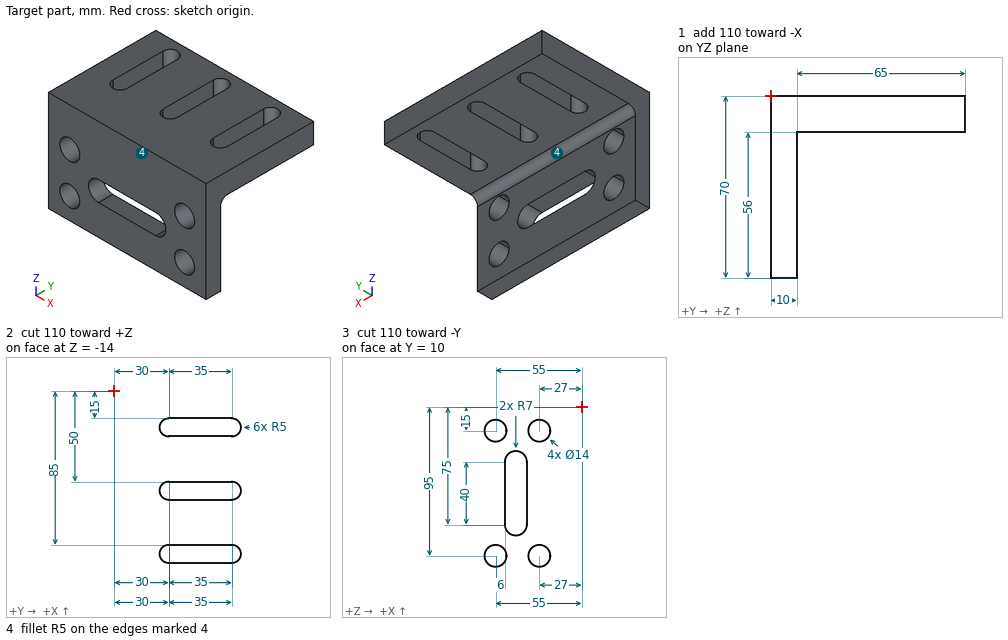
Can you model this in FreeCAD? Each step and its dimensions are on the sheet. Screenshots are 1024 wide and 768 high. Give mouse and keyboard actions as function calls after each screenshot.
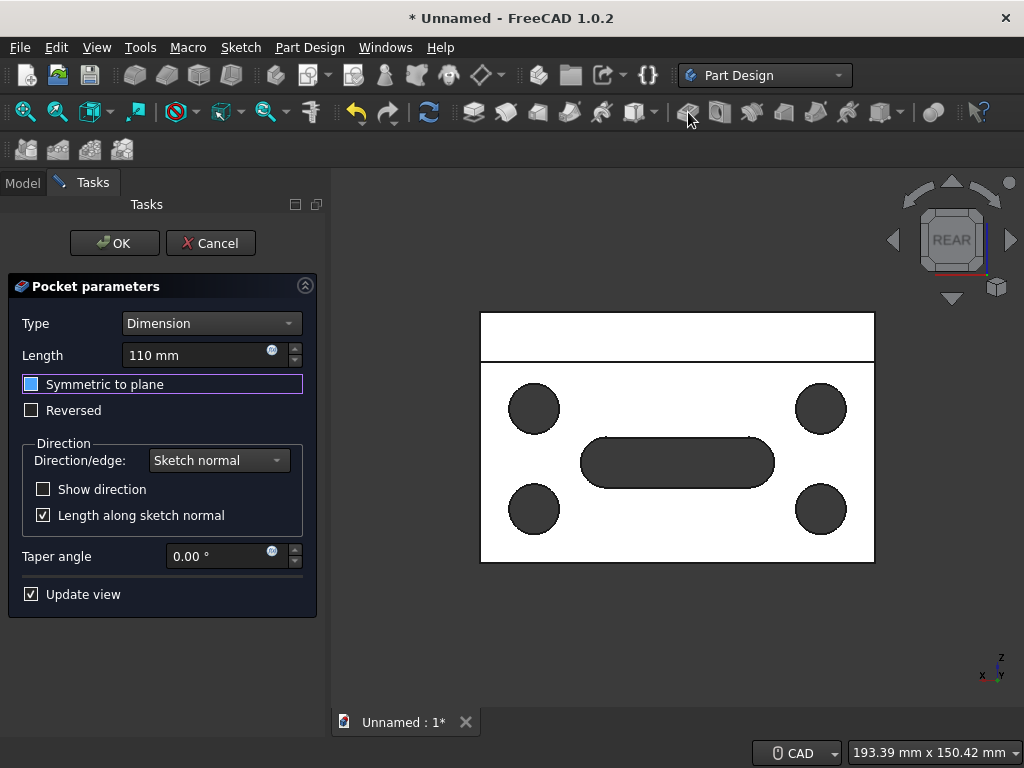
click(115, 243)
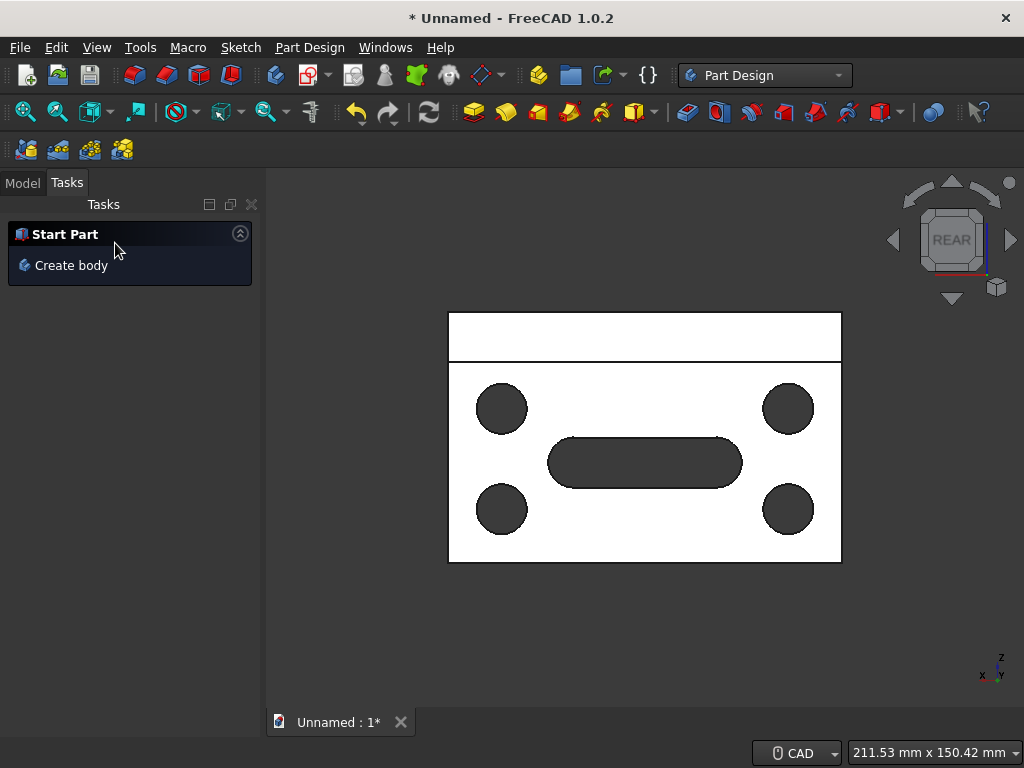
key(0)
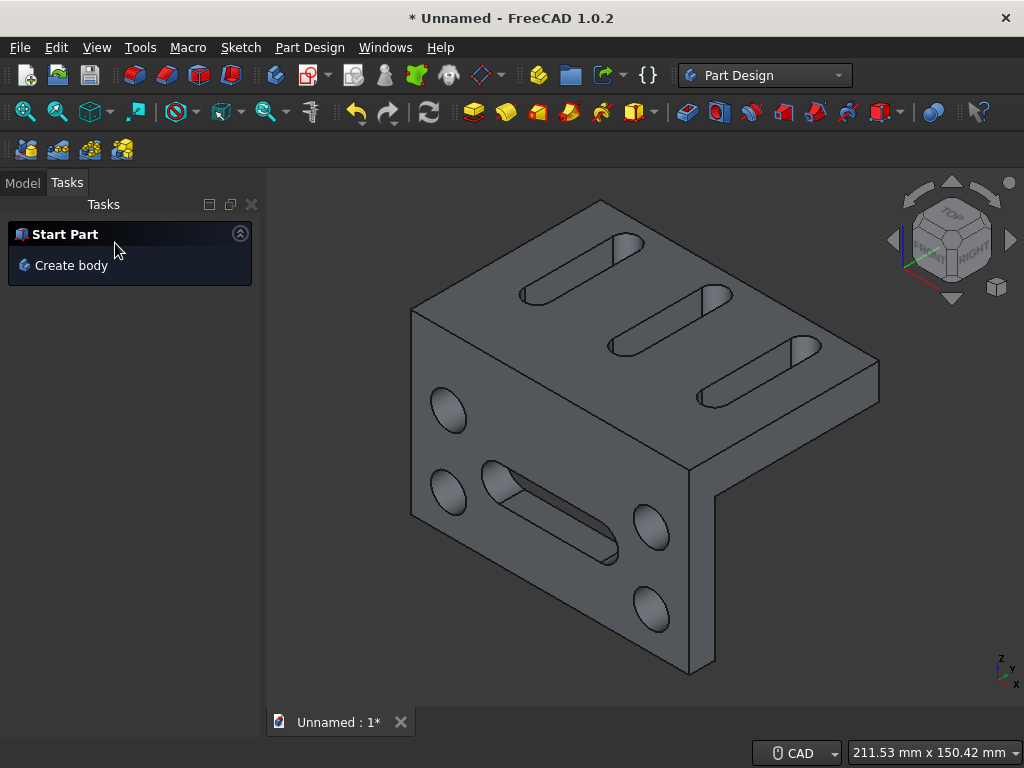
key(2)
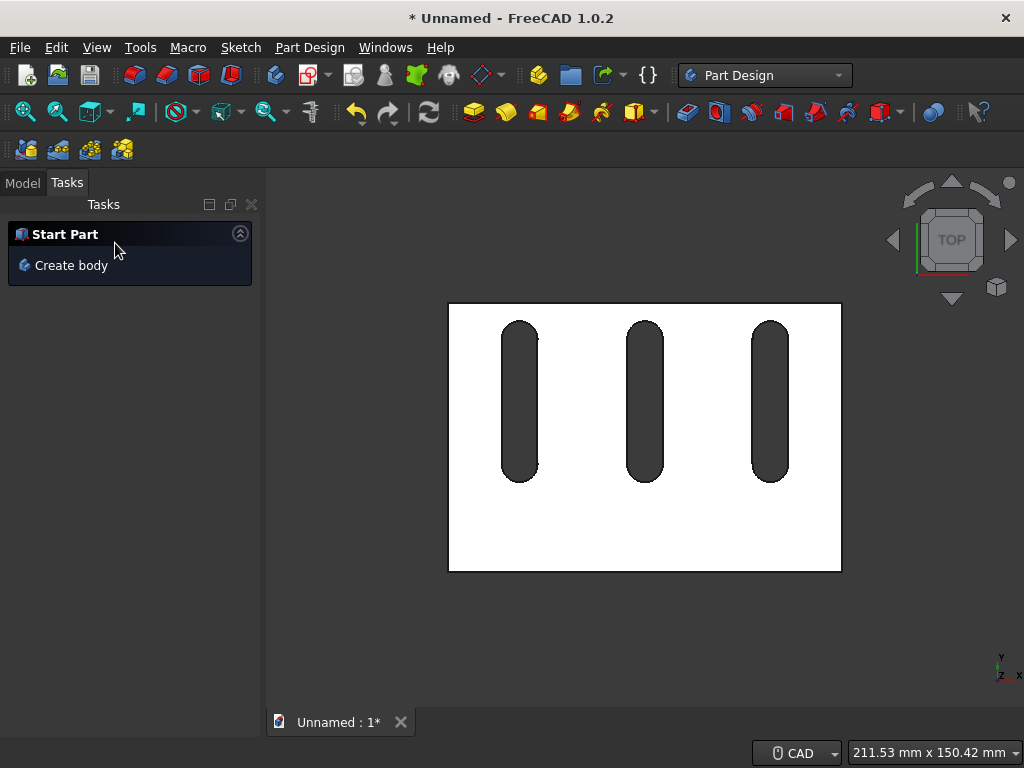
key(1)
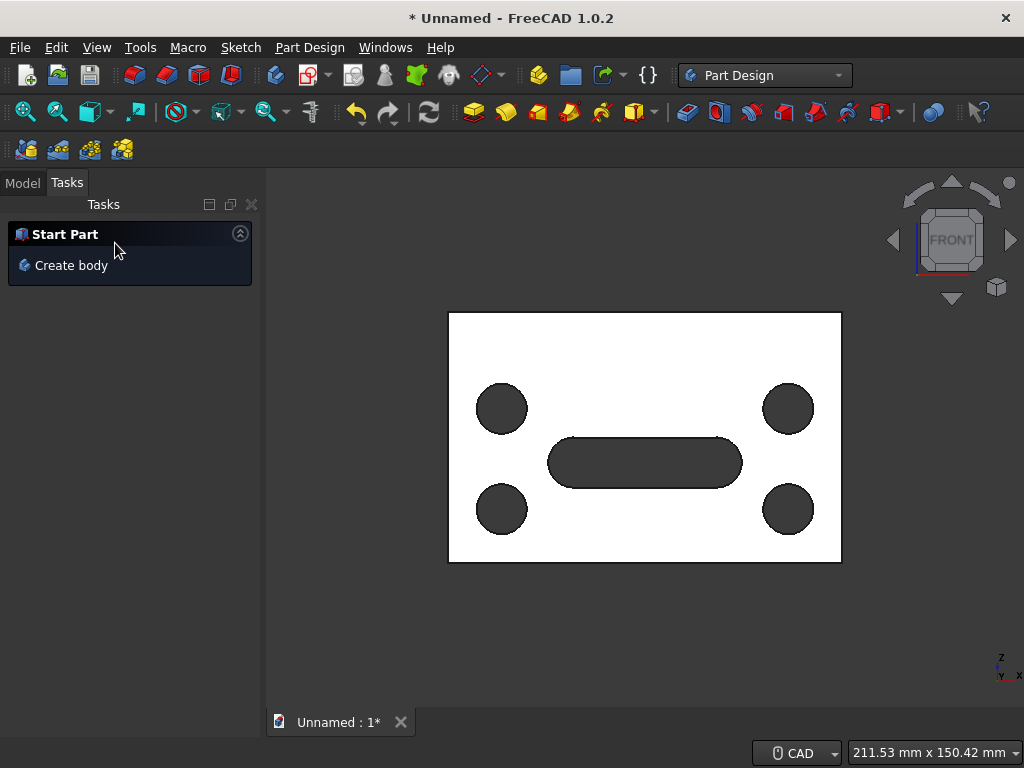
key(3)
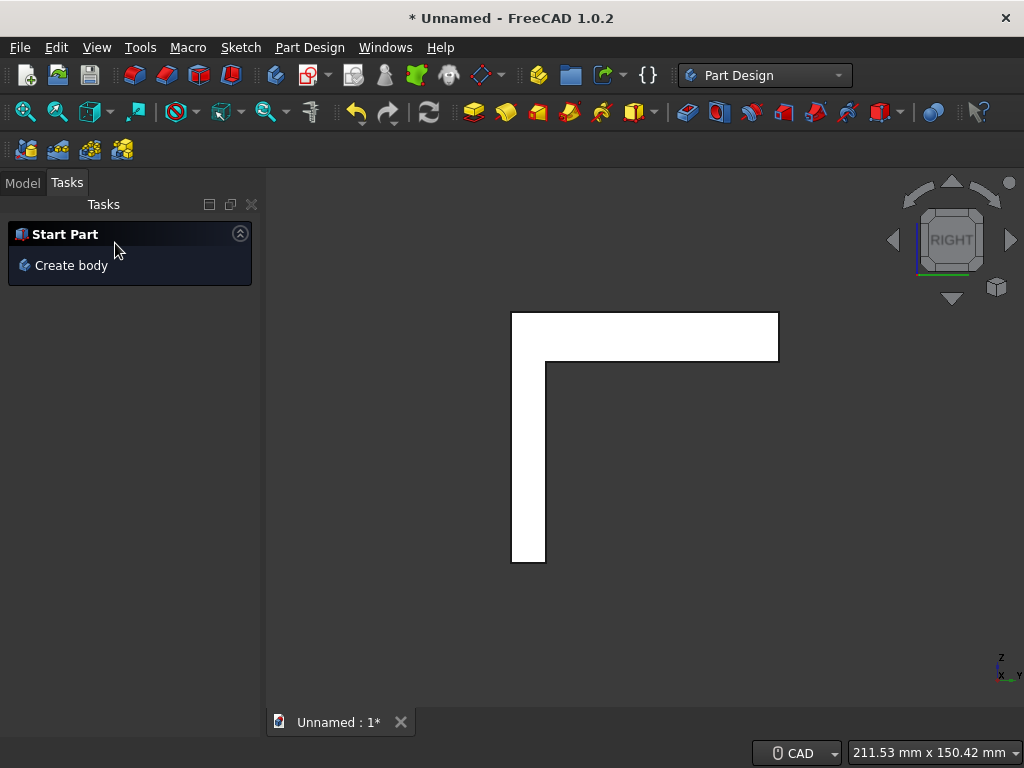
key(5)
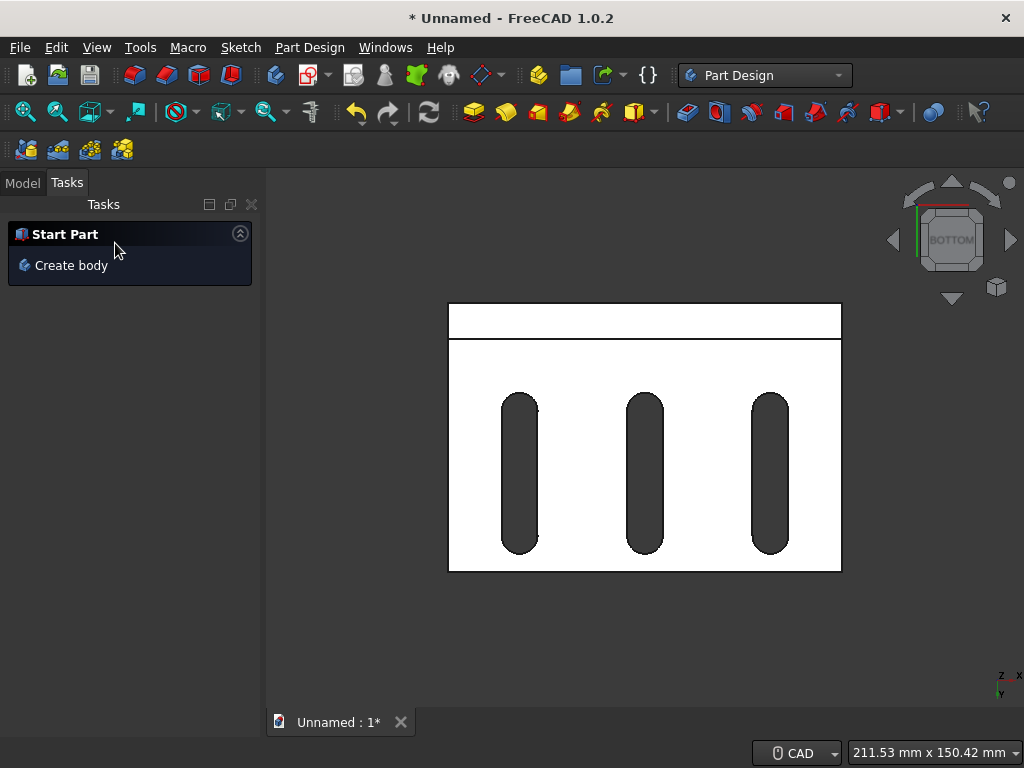
key(4)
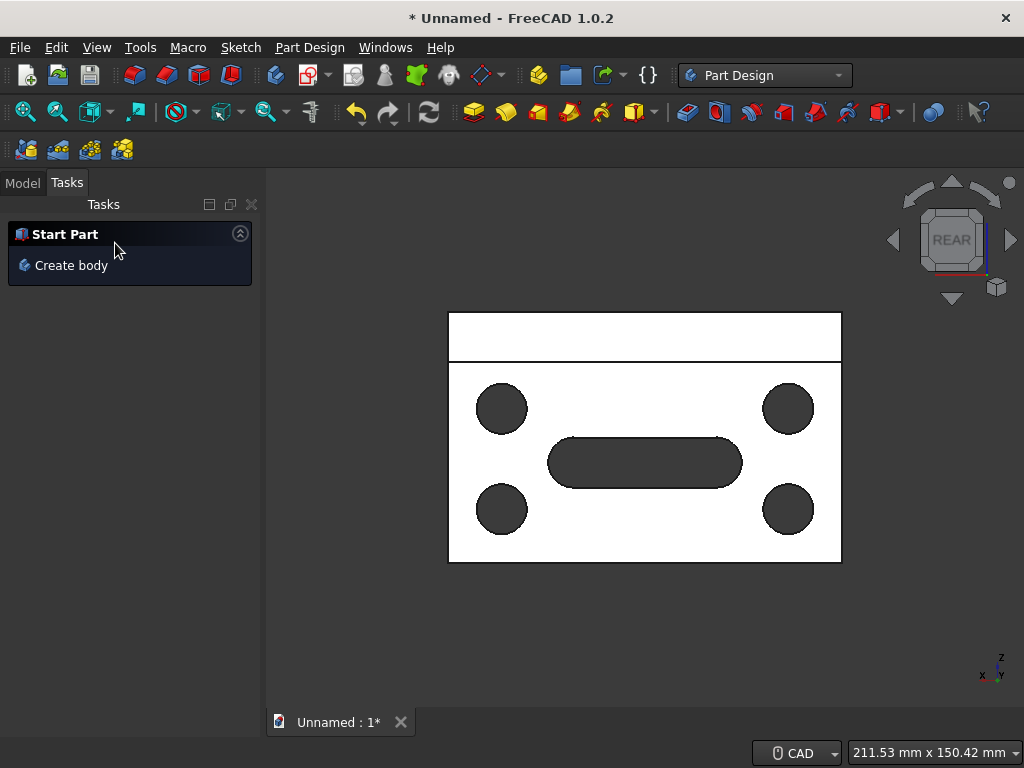
key(6)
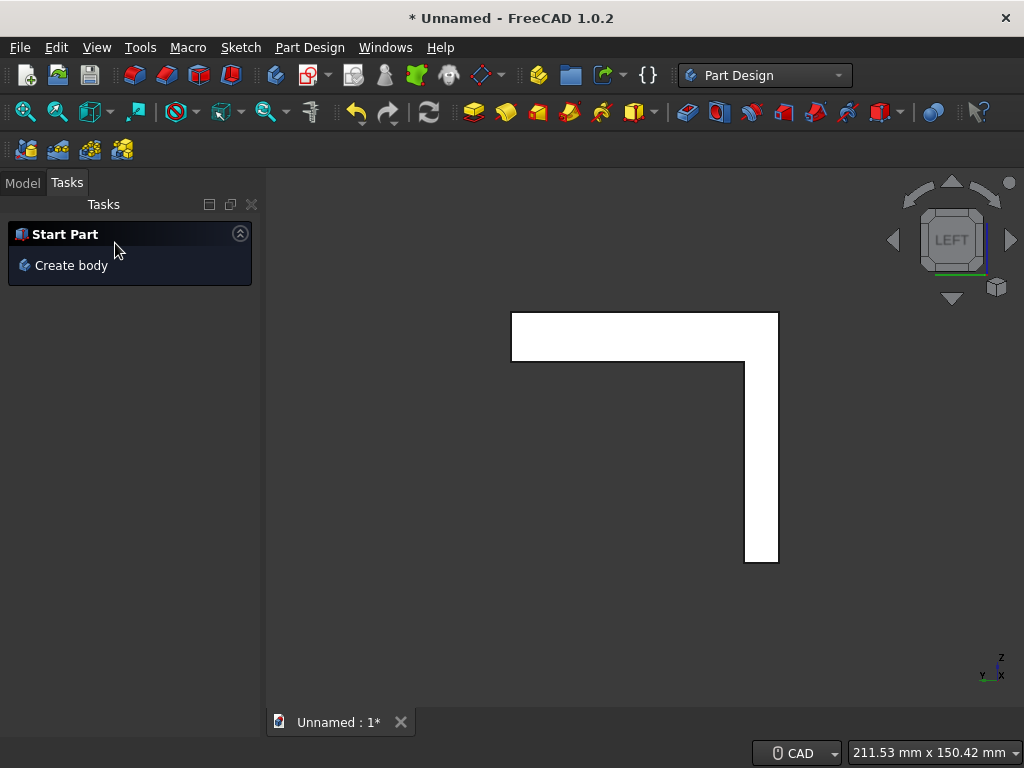
key(v)
key(3)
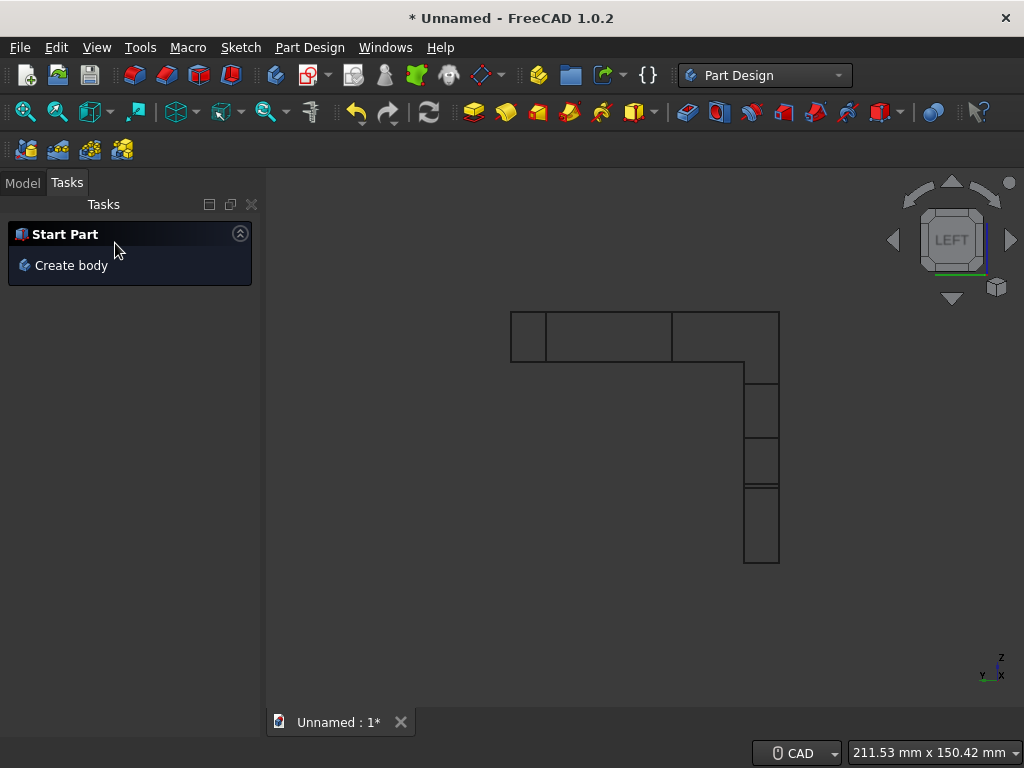
key(0)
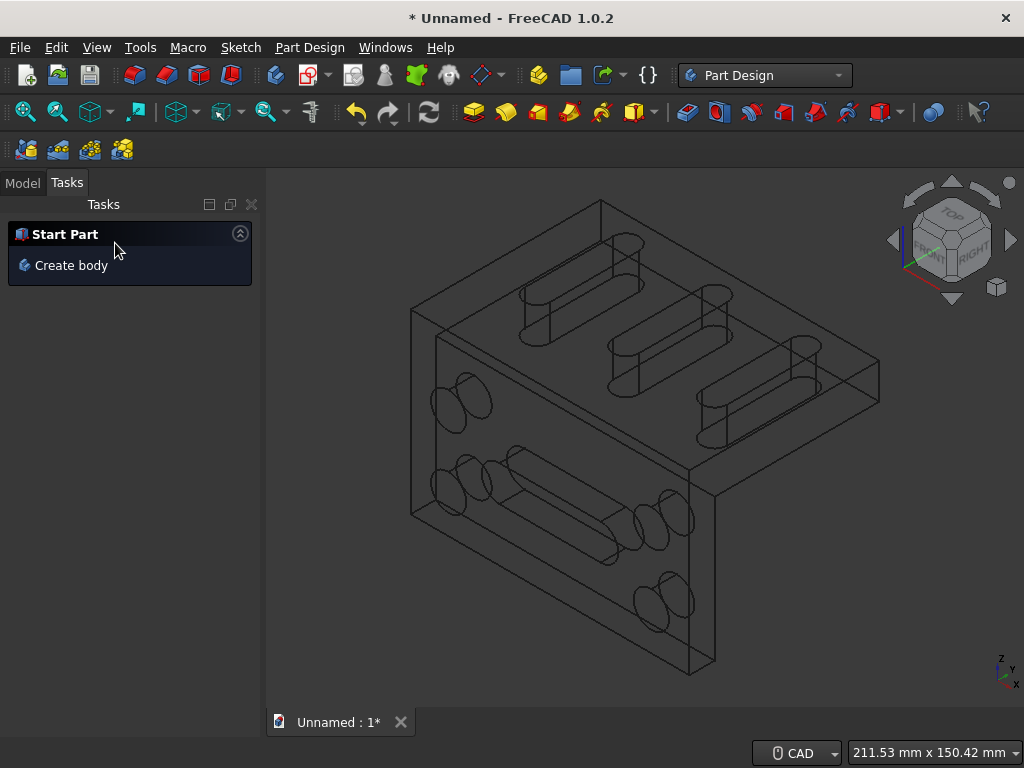
click(575, 415)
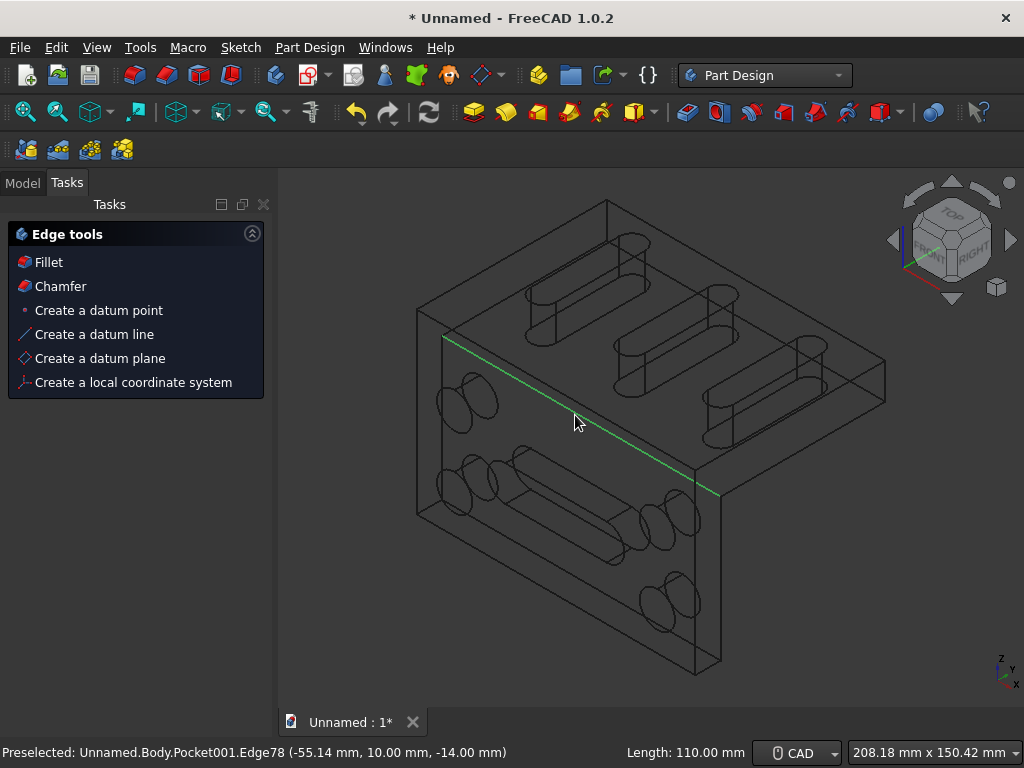
key(v)
key(1)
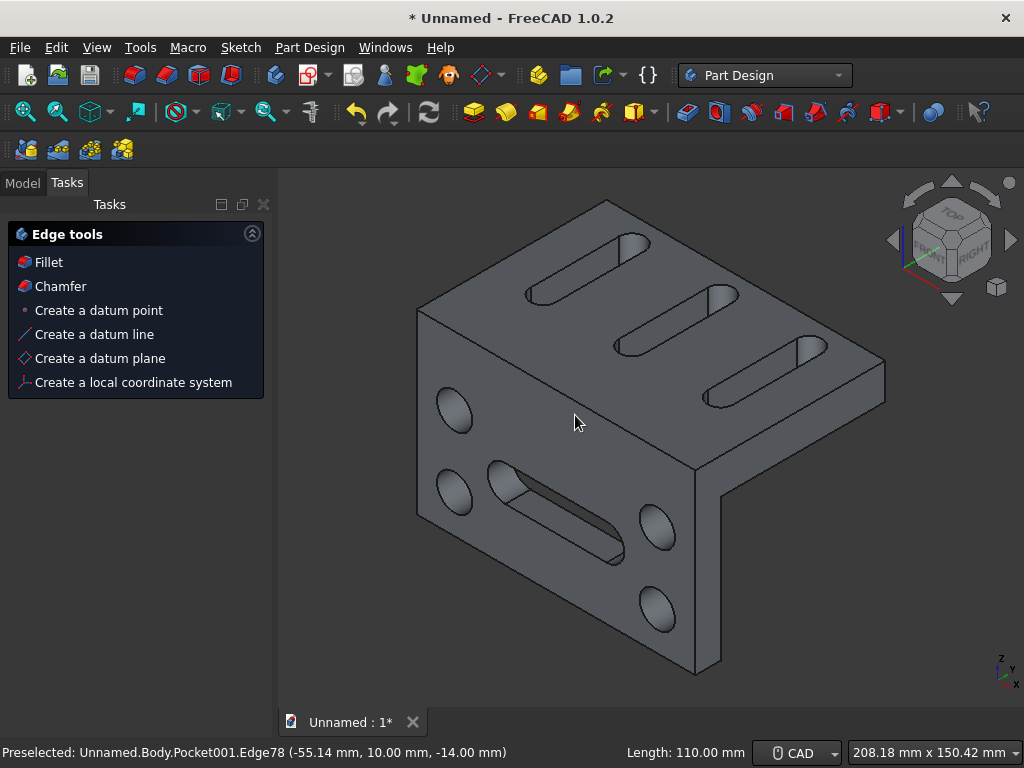
click(136, 76)